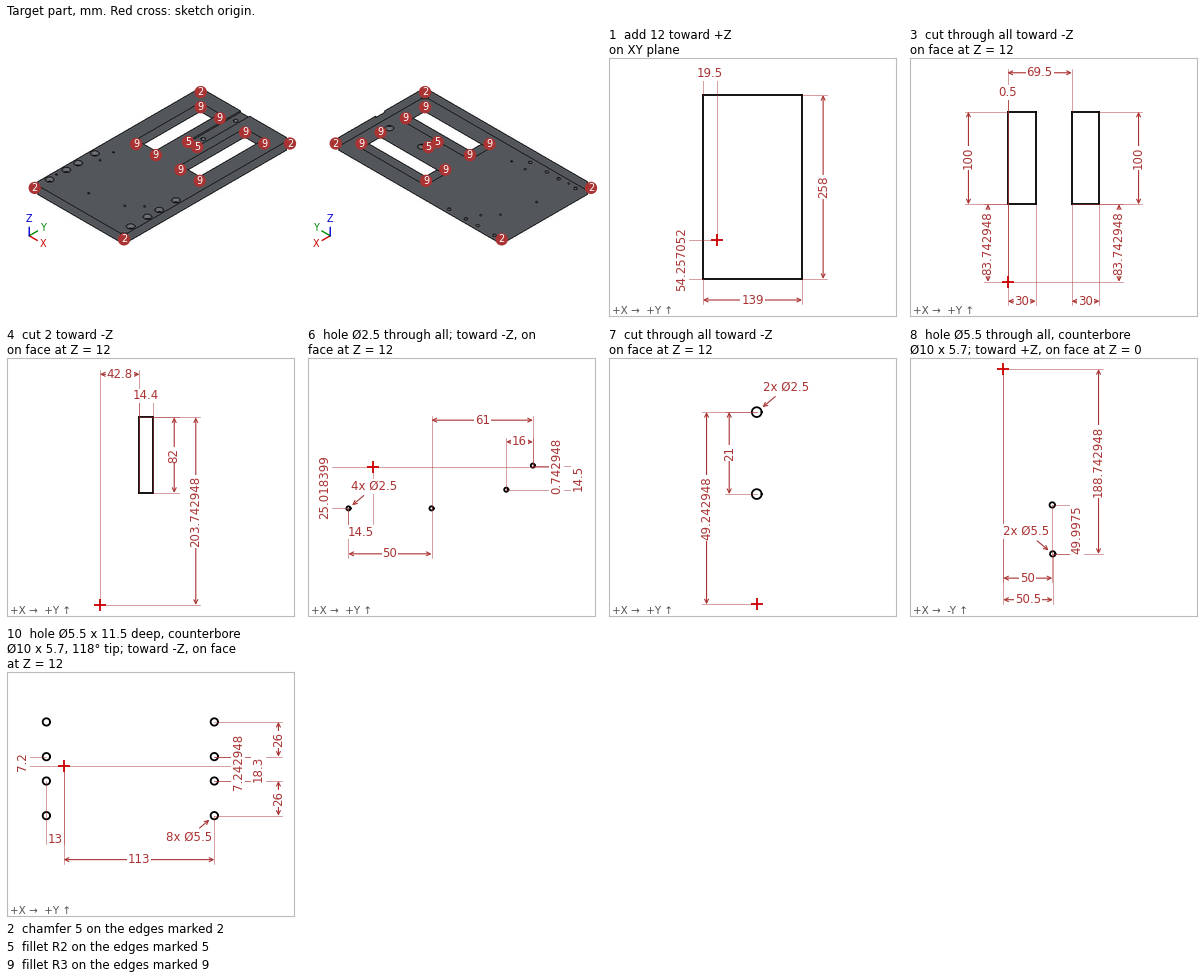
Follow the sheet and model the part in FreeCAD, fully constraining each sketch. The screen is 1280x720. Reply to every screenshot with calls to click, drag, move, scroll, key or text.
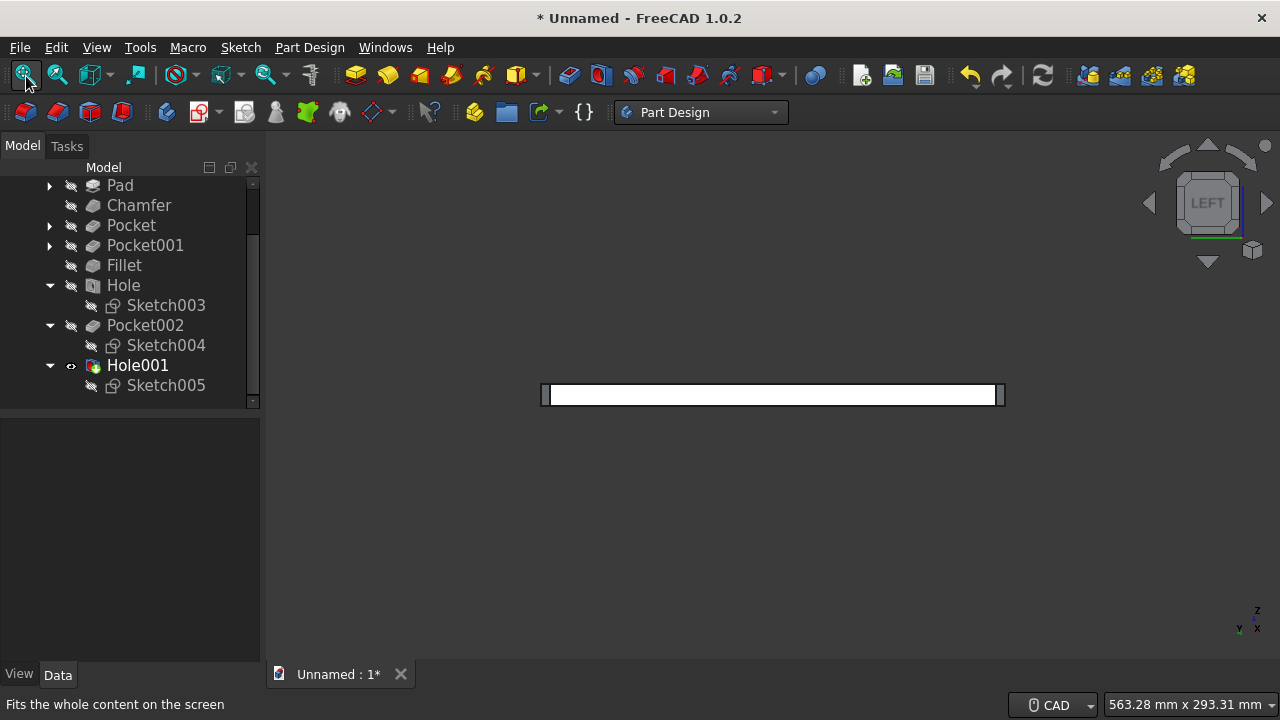
key(v)
key(3)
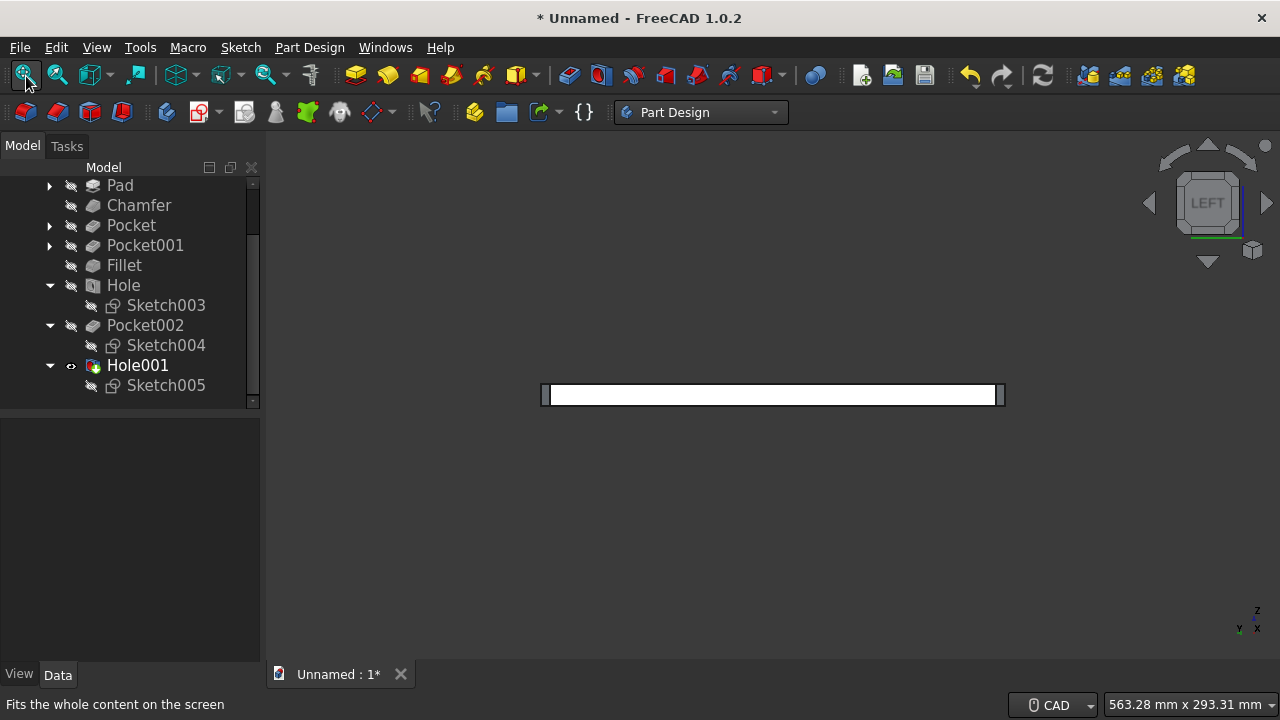
key(0)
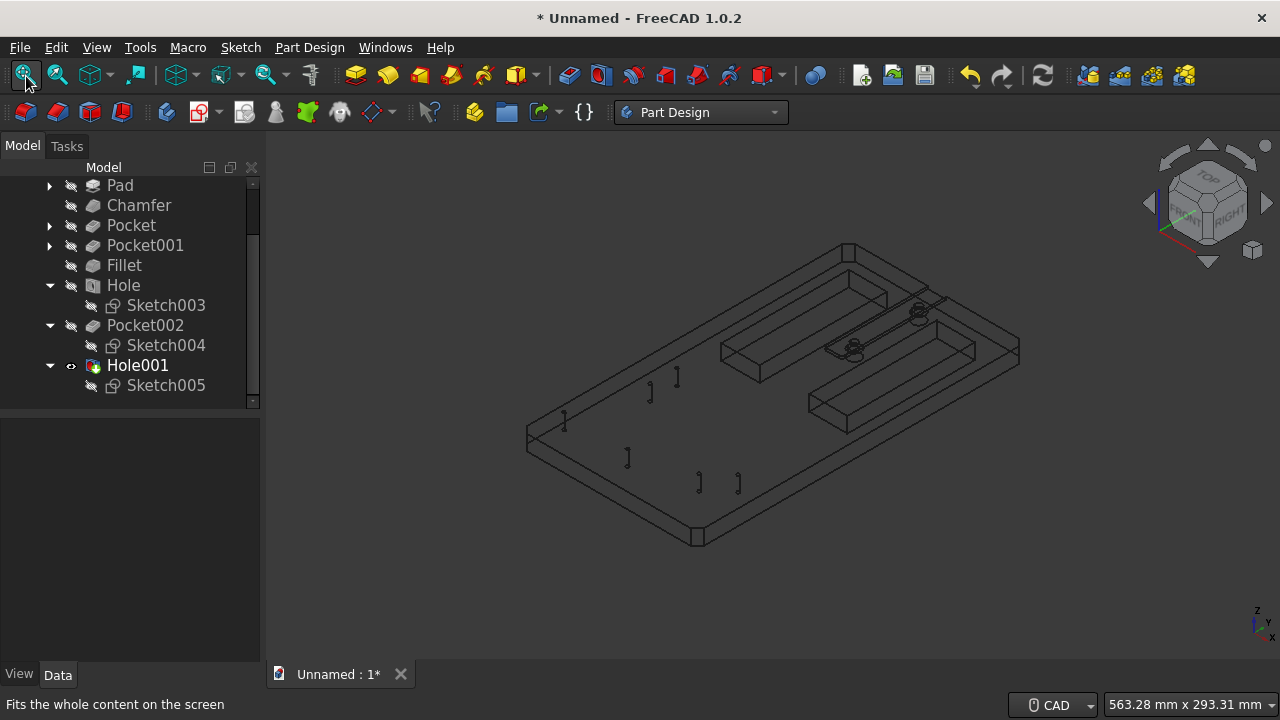
click(975, 350)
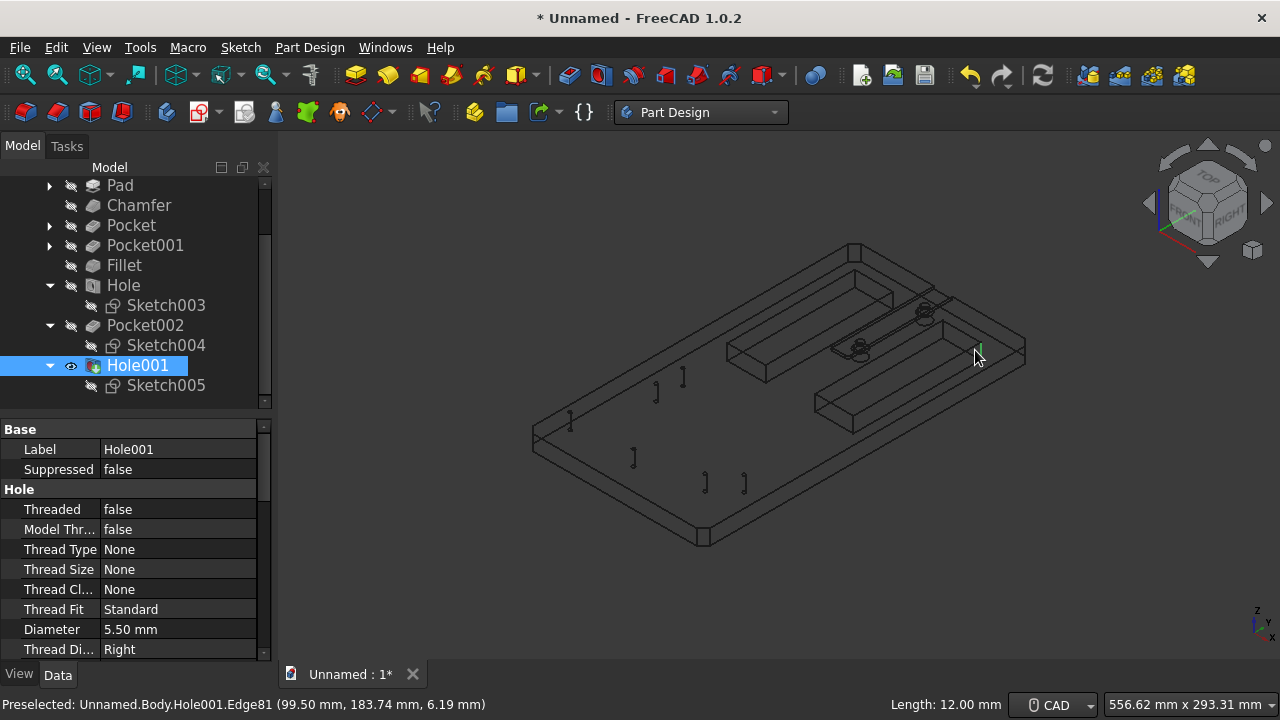
click(853, 424, ctrl)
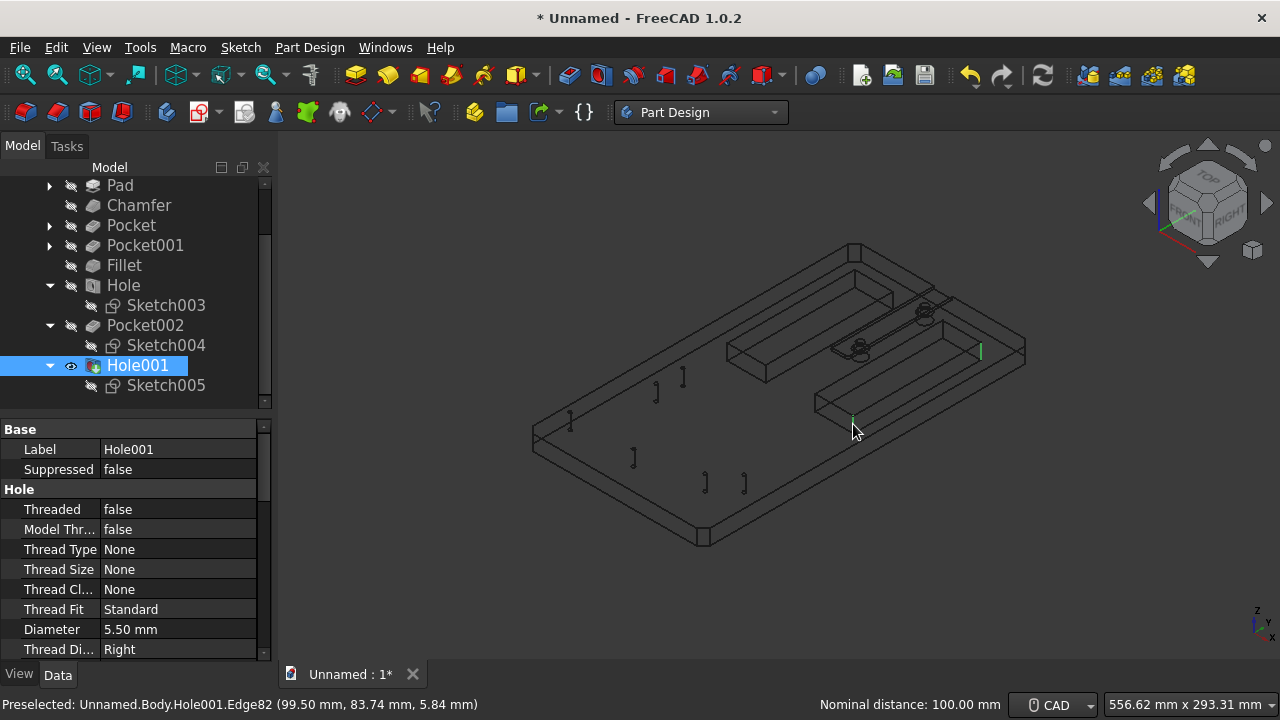
click(815, 402, ctrl)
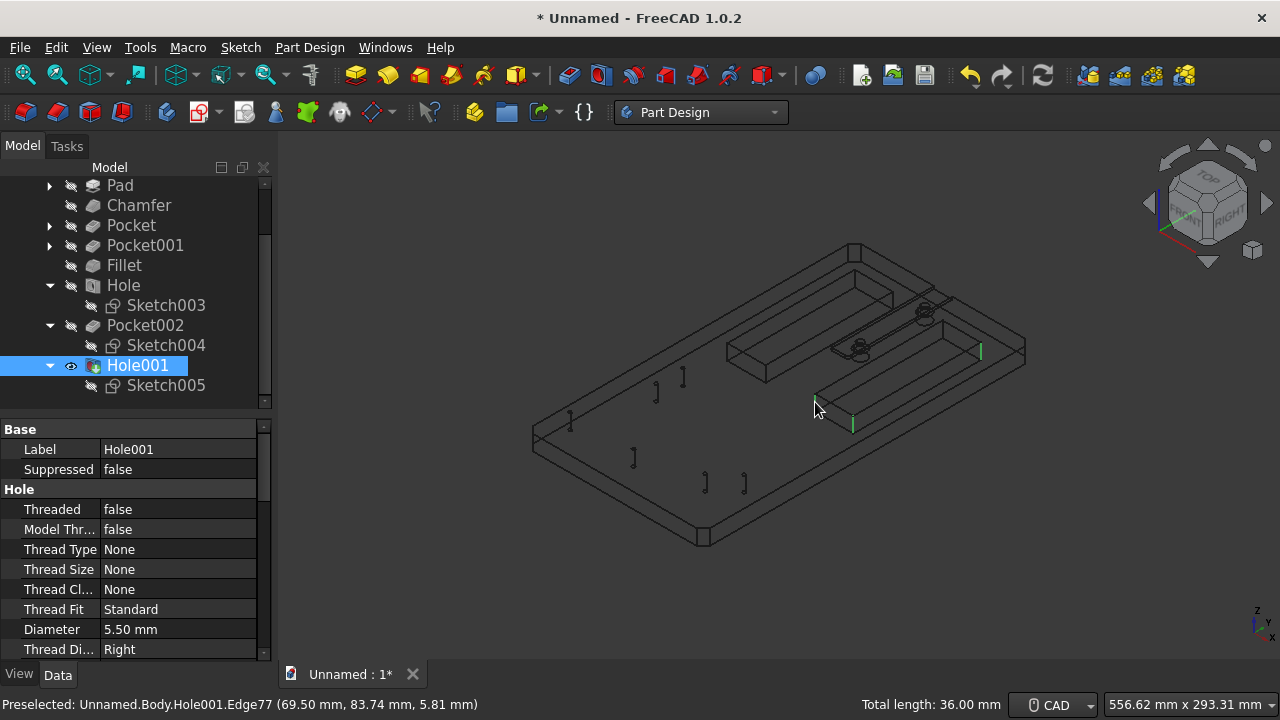
click(943, 328, ctrl)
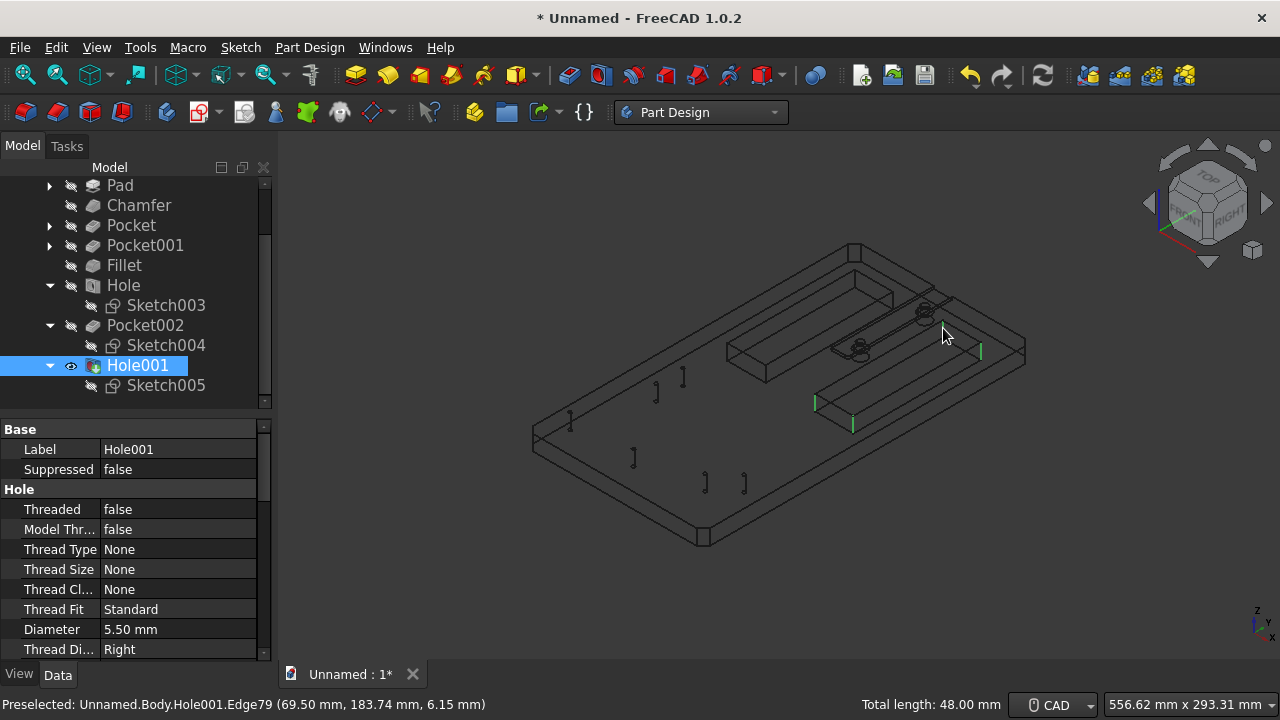
click(766, 373, ctrl)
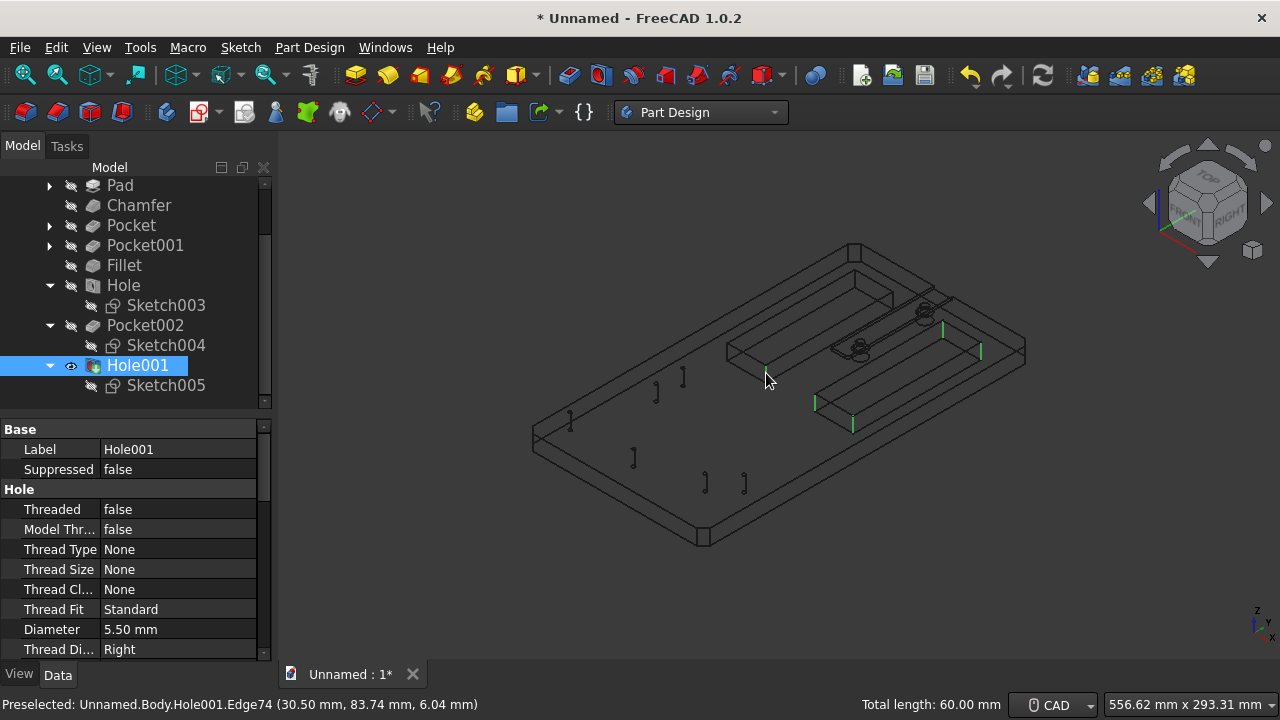
click(727, 351, ctrl)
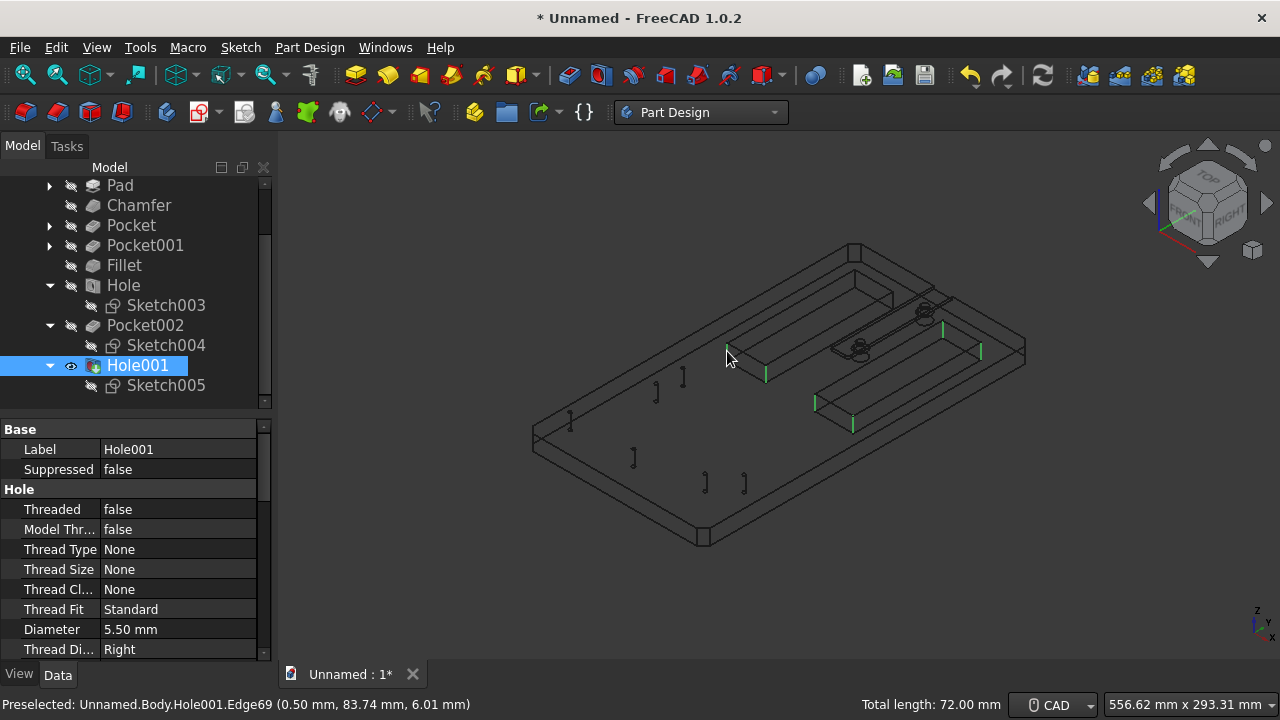
click(855, 278, ctrl)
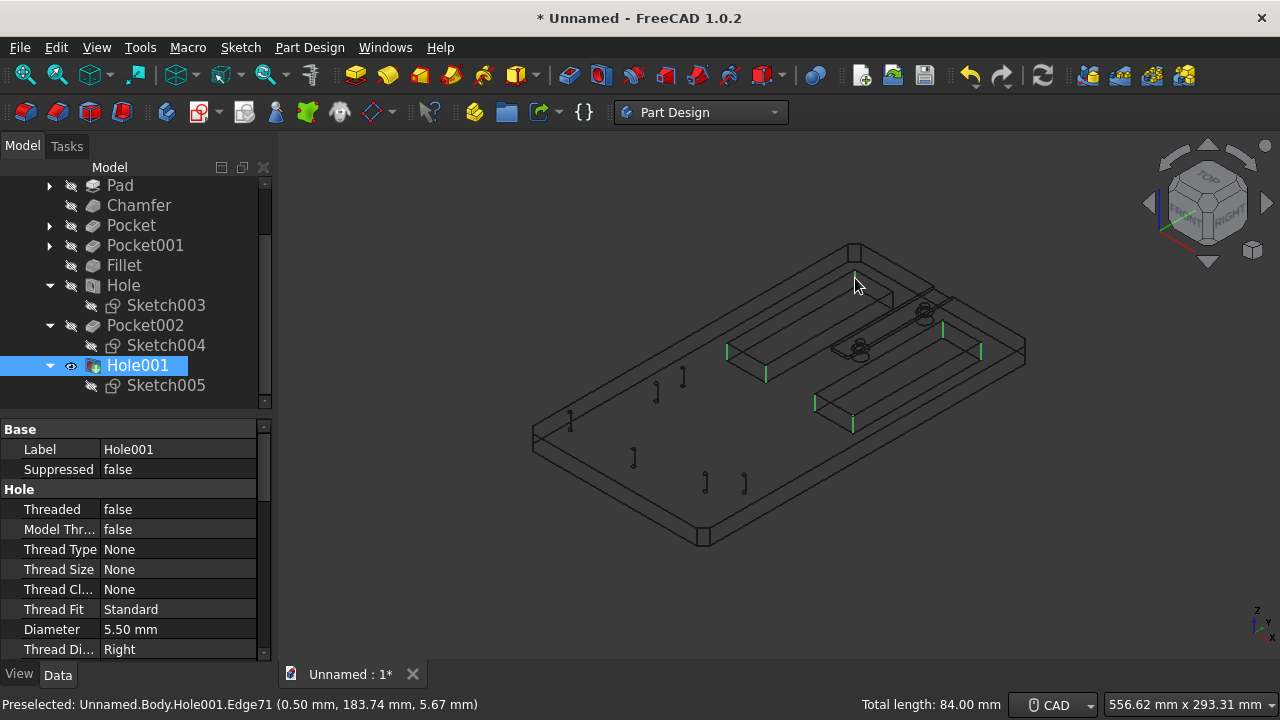
click(893, 300, ctrl)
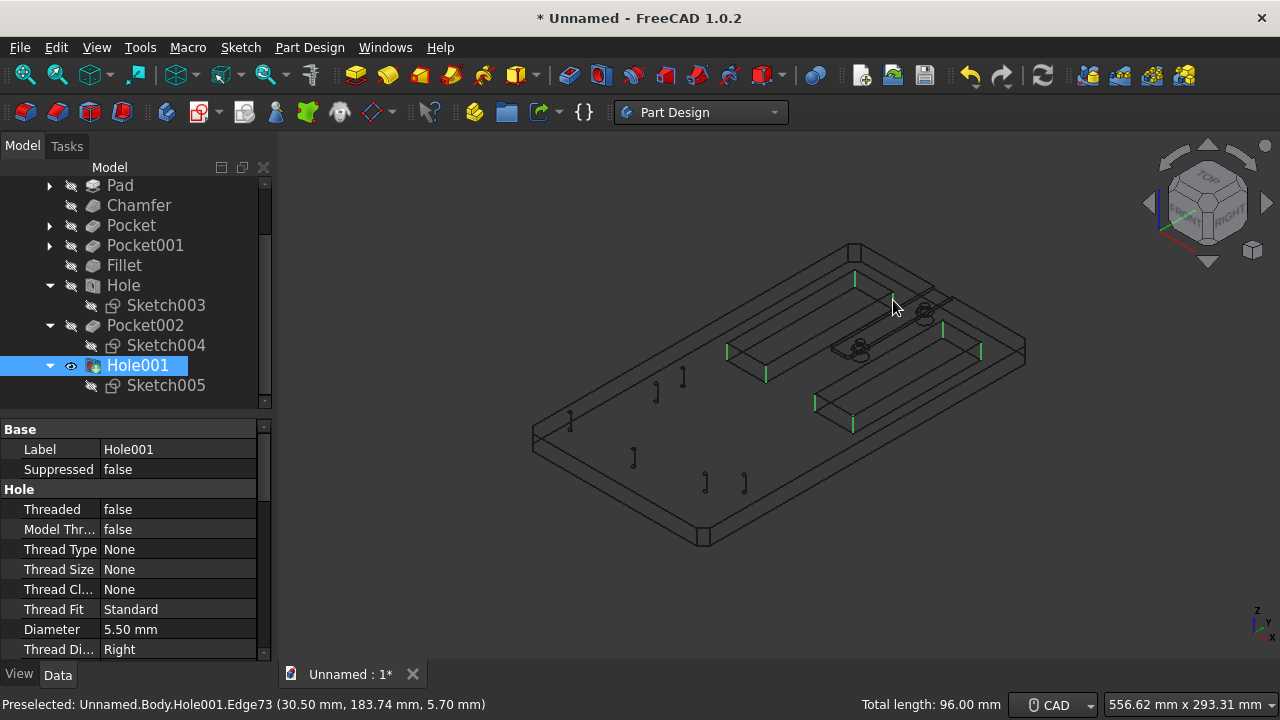
key(v)
key(1)